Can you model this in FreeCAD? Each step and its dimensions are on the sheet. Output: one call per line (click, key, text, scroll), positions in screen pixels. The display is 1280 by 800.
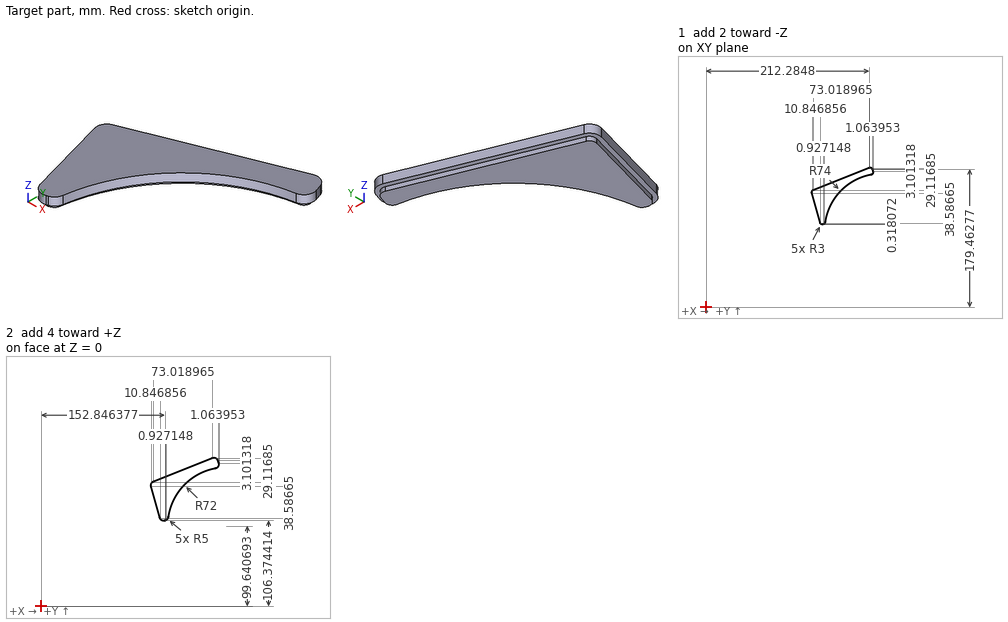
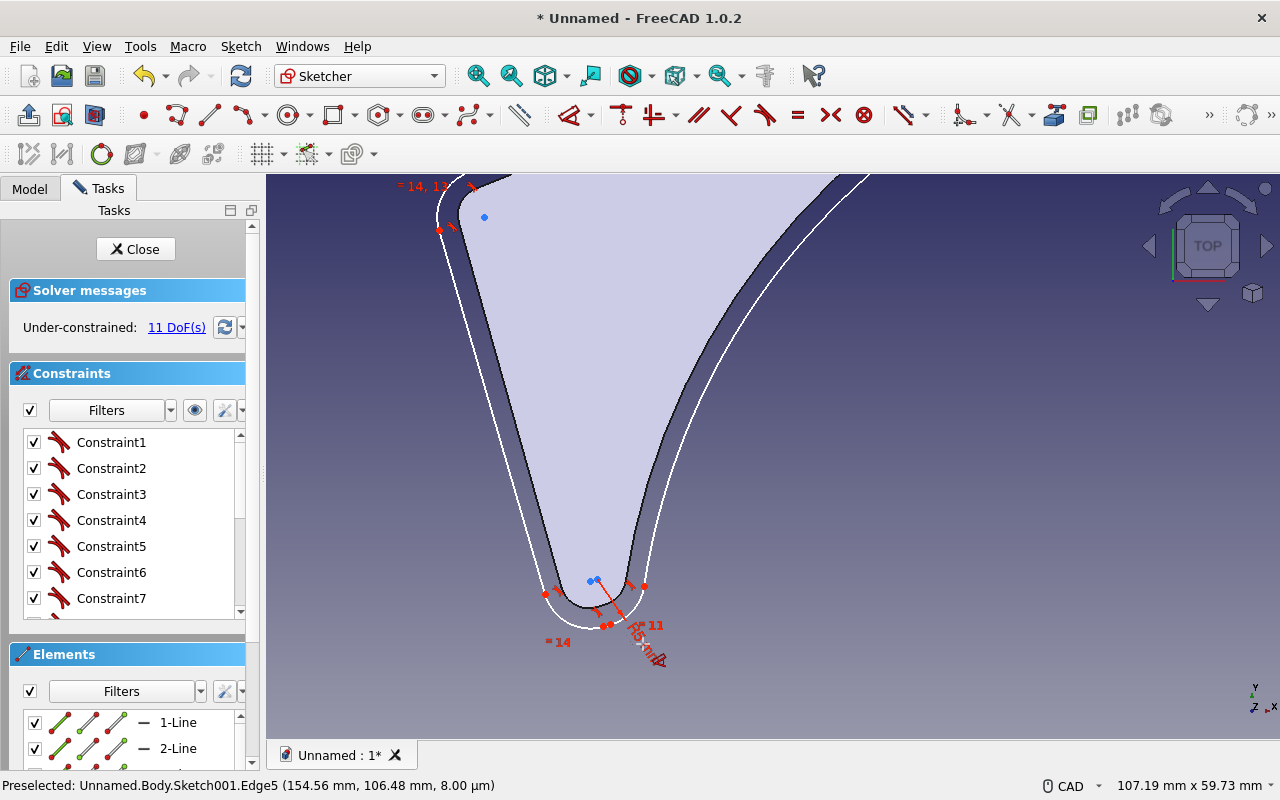
click(727, 348)
click(699, 332)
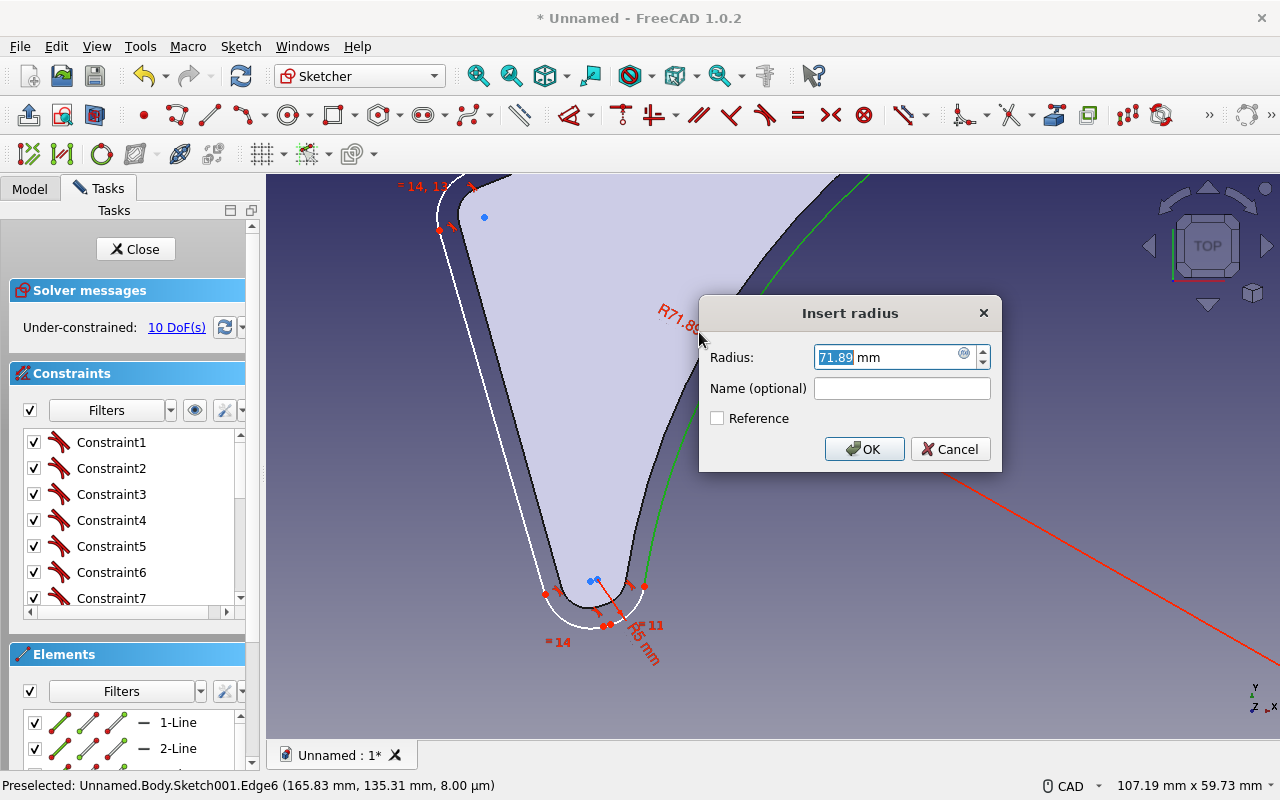
text(72)
key(Return)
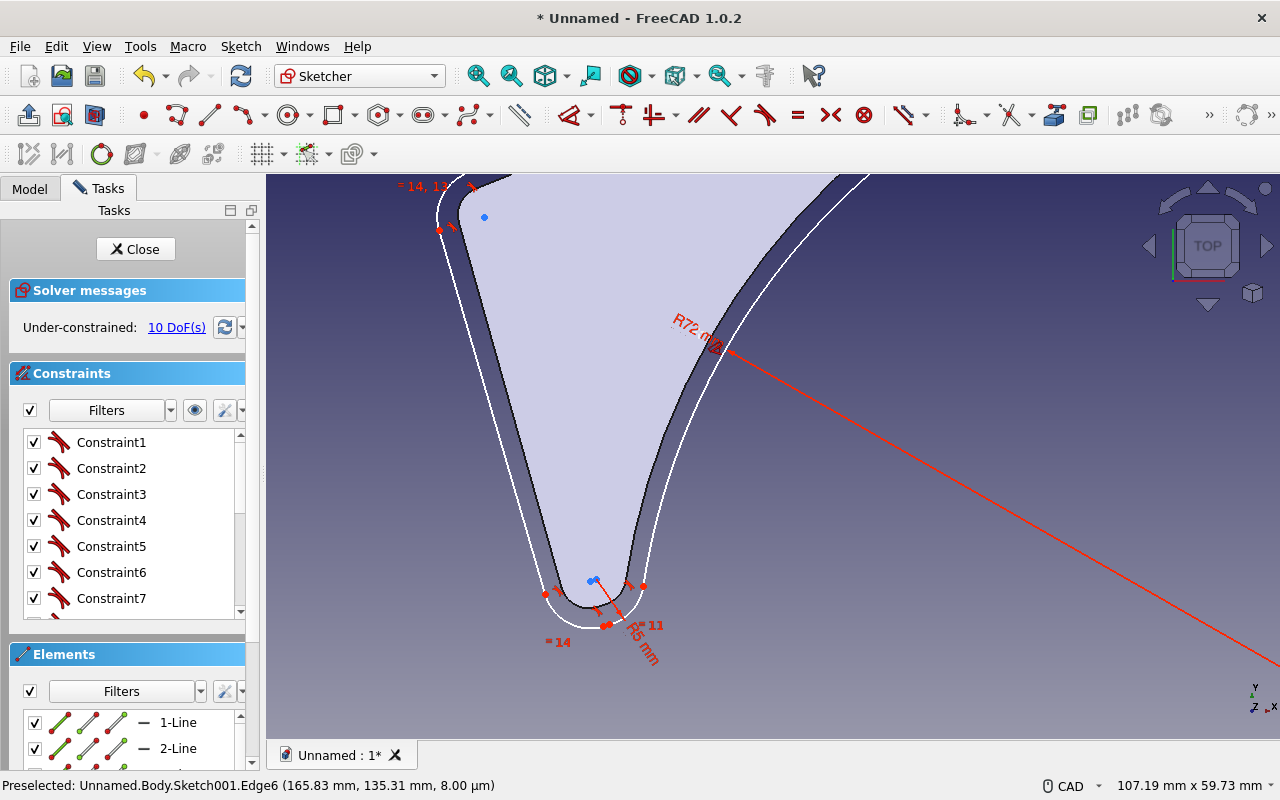
scroll(607, 626, up, 8)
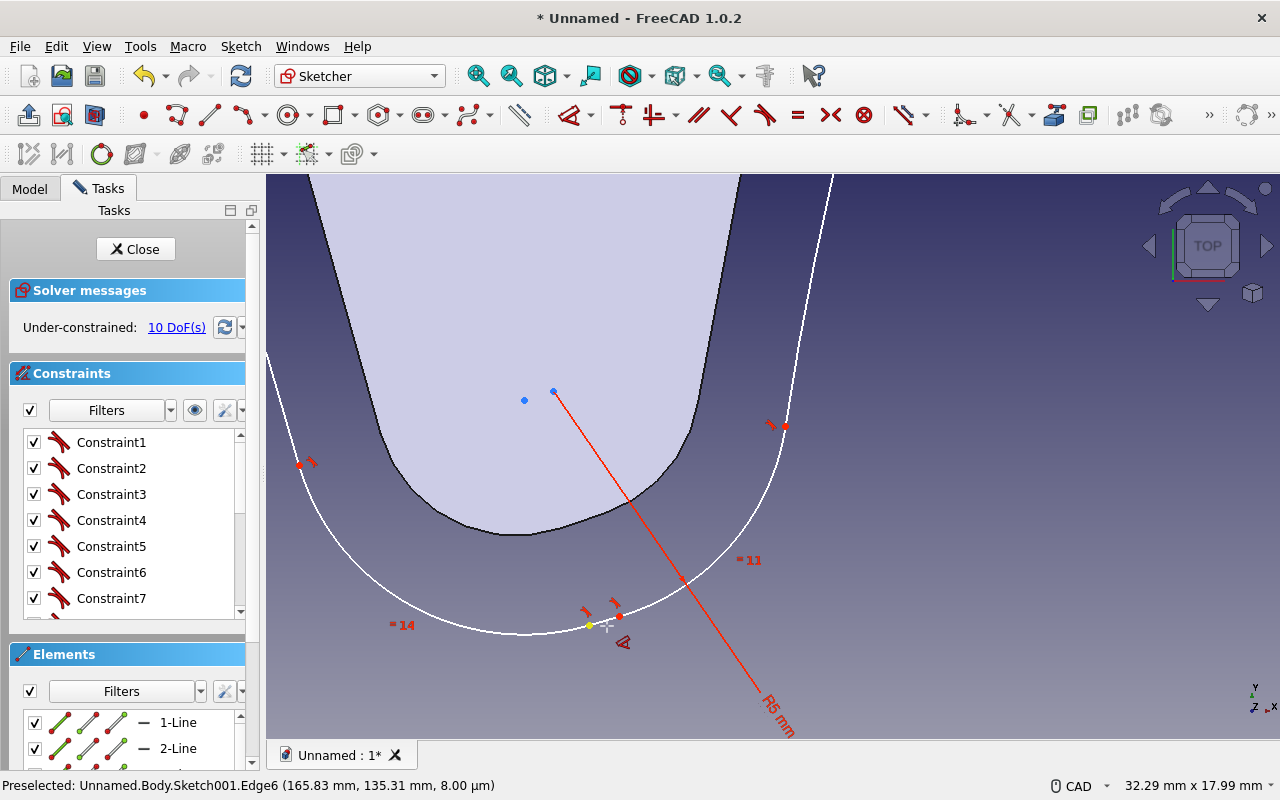
click(605, 621)
click(605, 659)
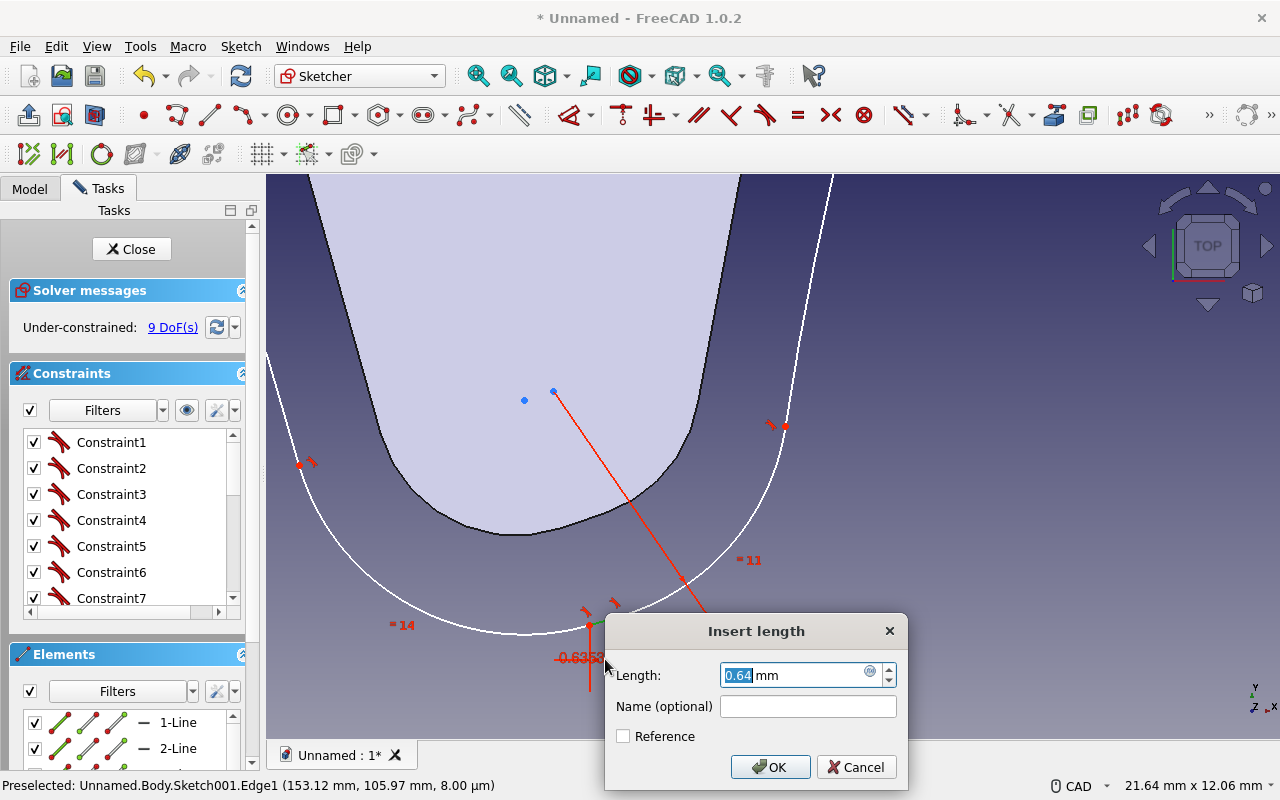
text(0.927148)
key(Return)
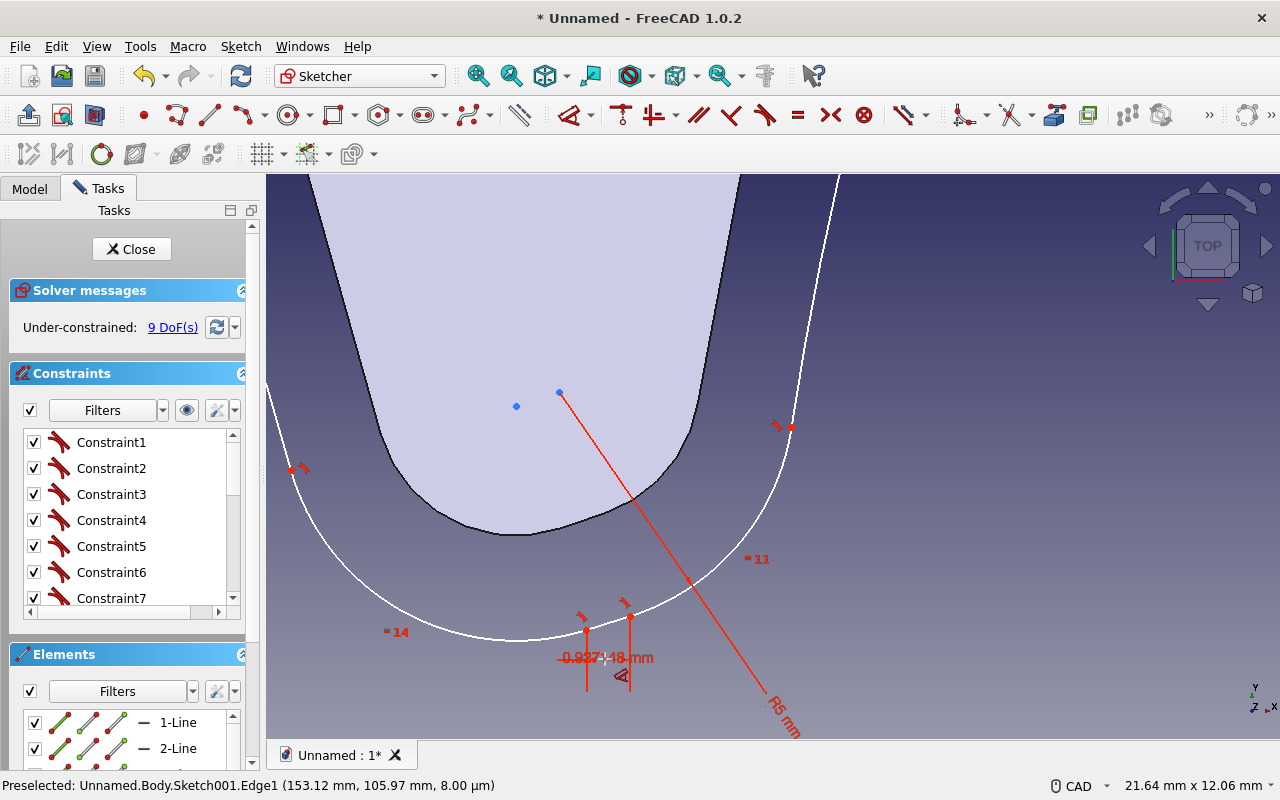
scroll(601, 621, down, 12)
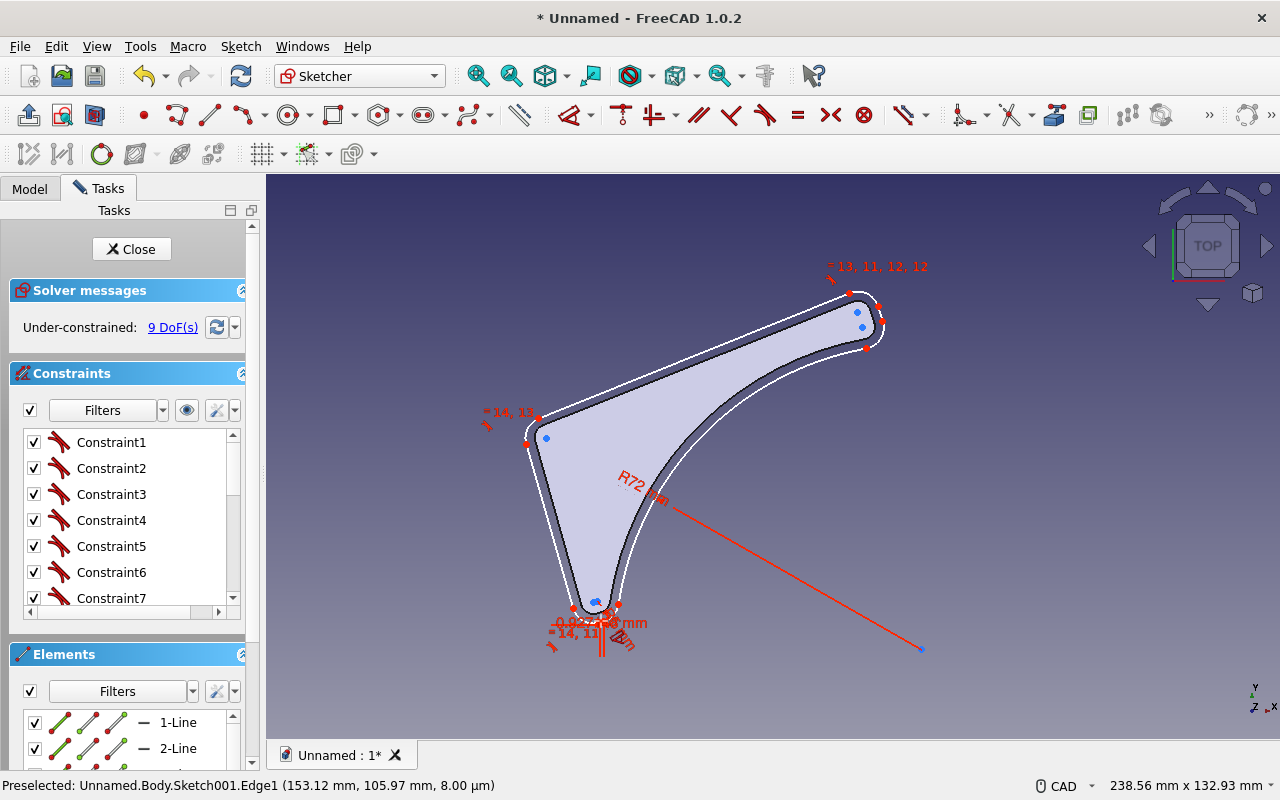
scroll(881, 317, up, 11)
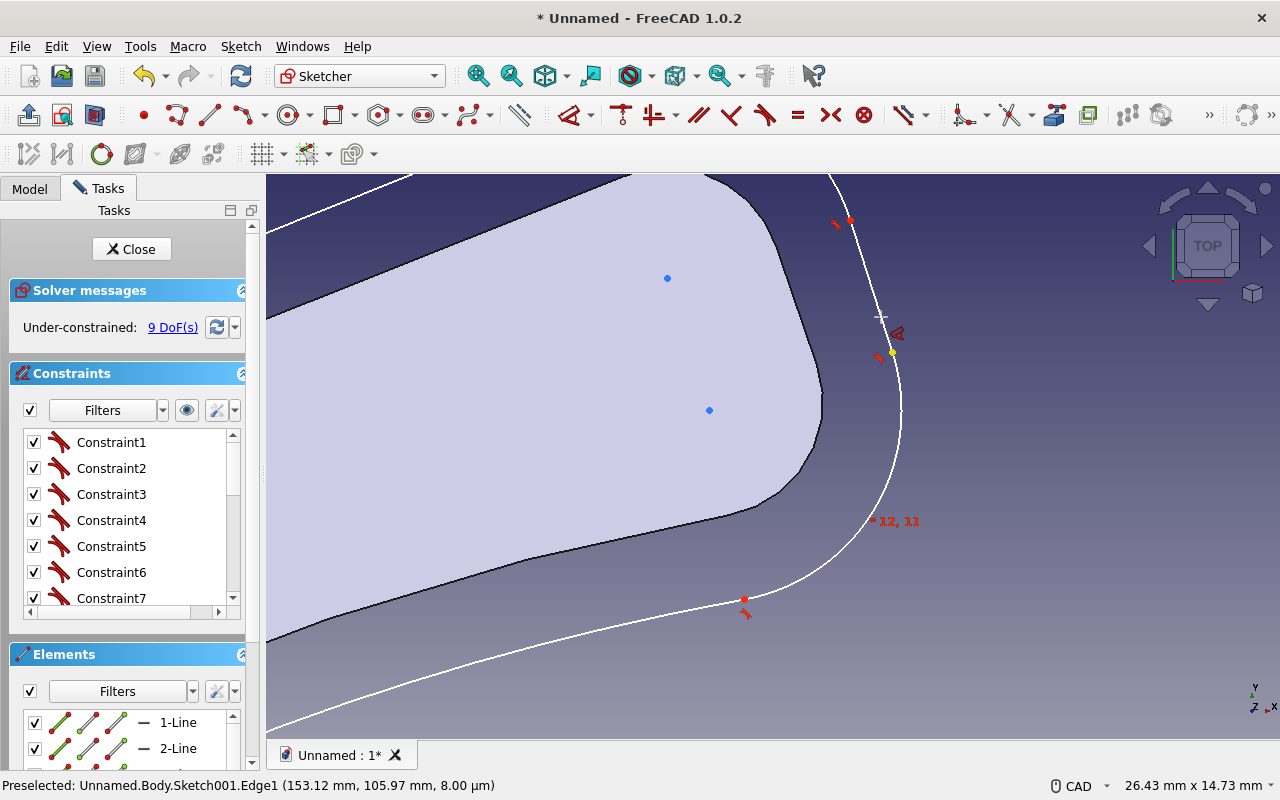
click(880, 313)
click(871, 387)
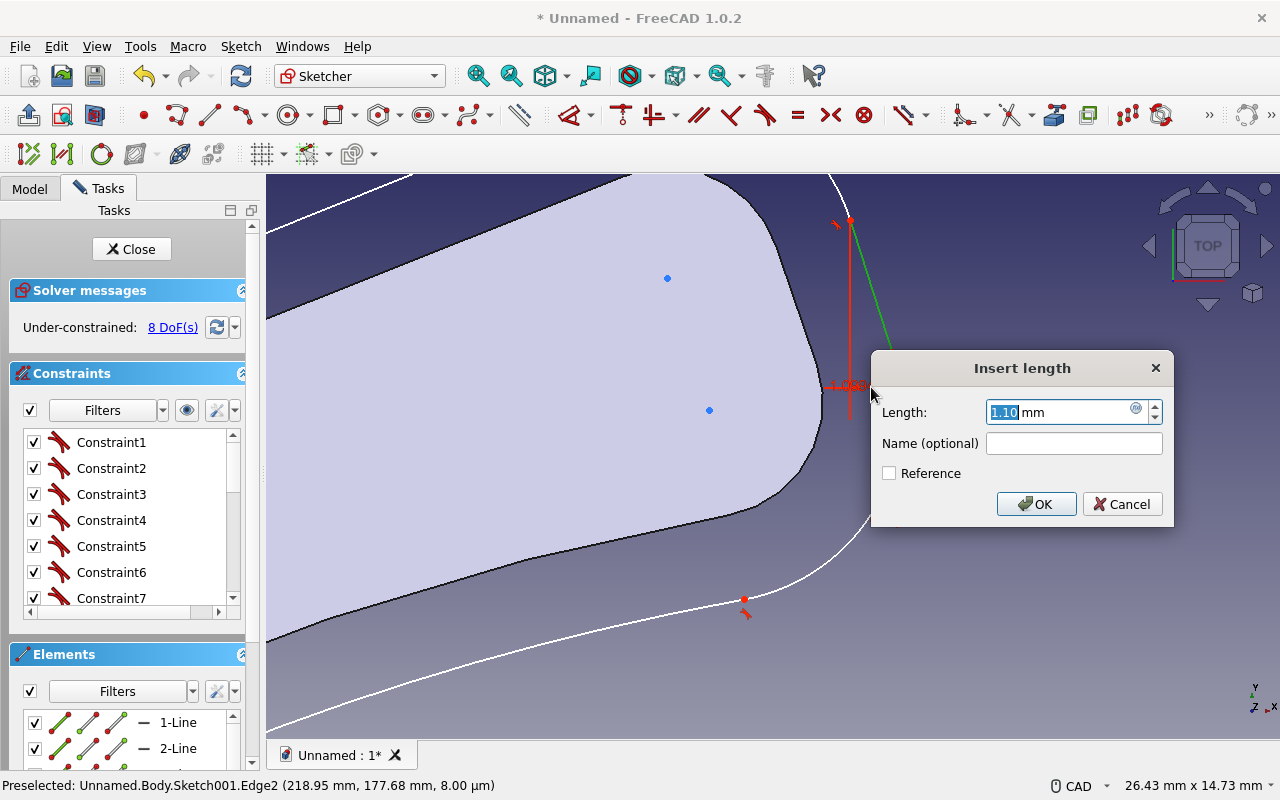
text(1.063953)
key(Return)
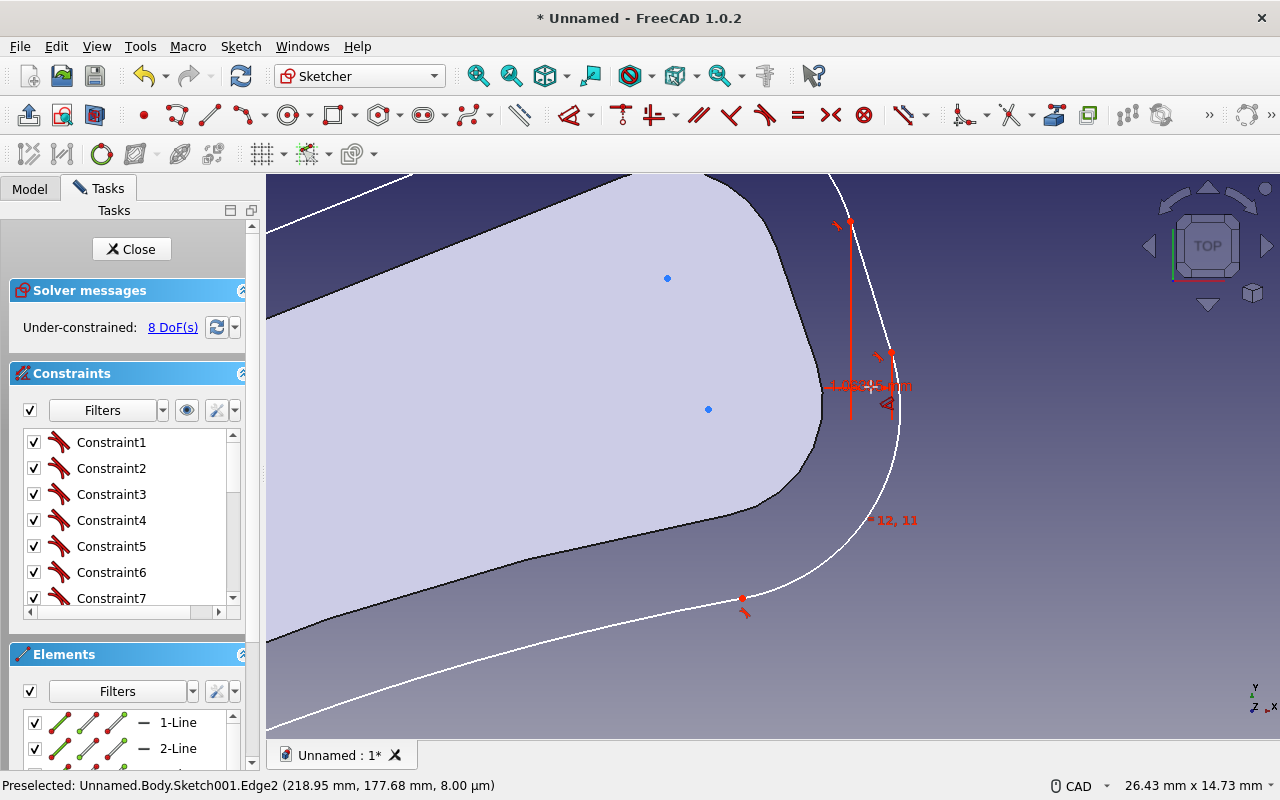
scroll(881, 316, down, 11)